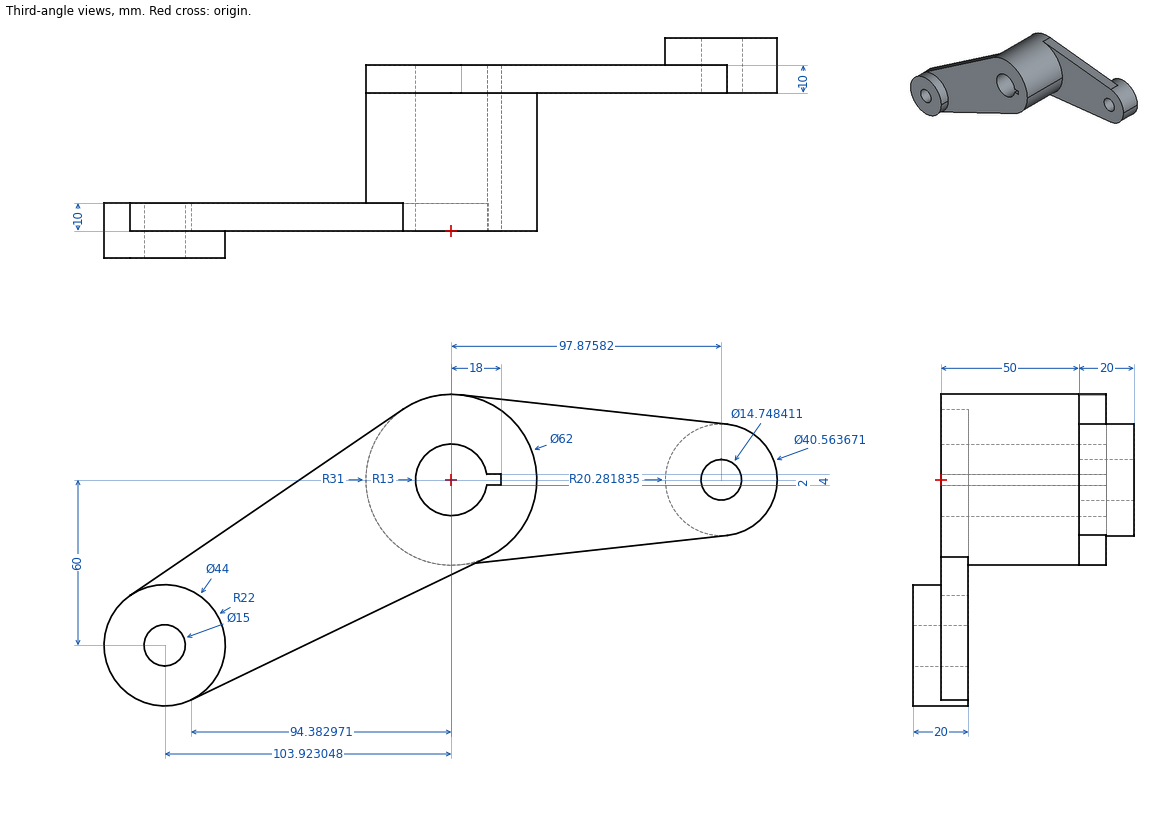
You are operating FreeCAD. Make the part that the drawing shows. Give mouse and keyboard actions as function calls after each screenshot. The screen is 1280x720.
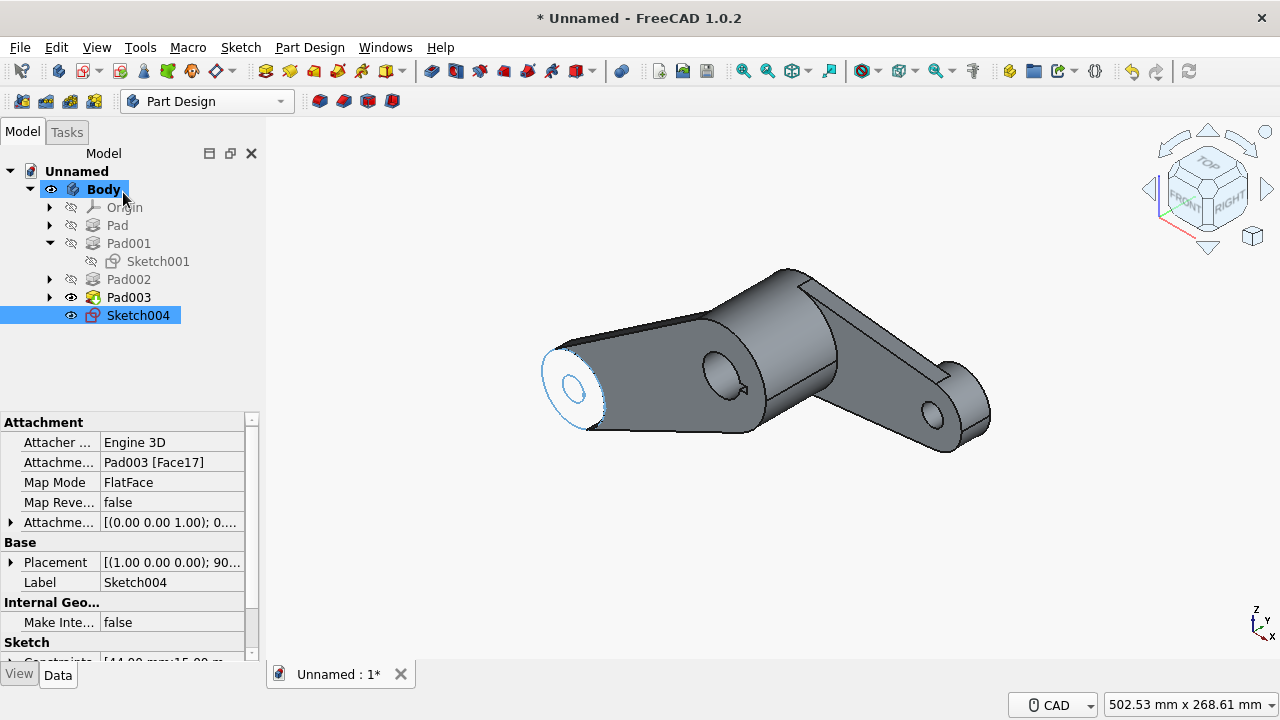
click(266, 72)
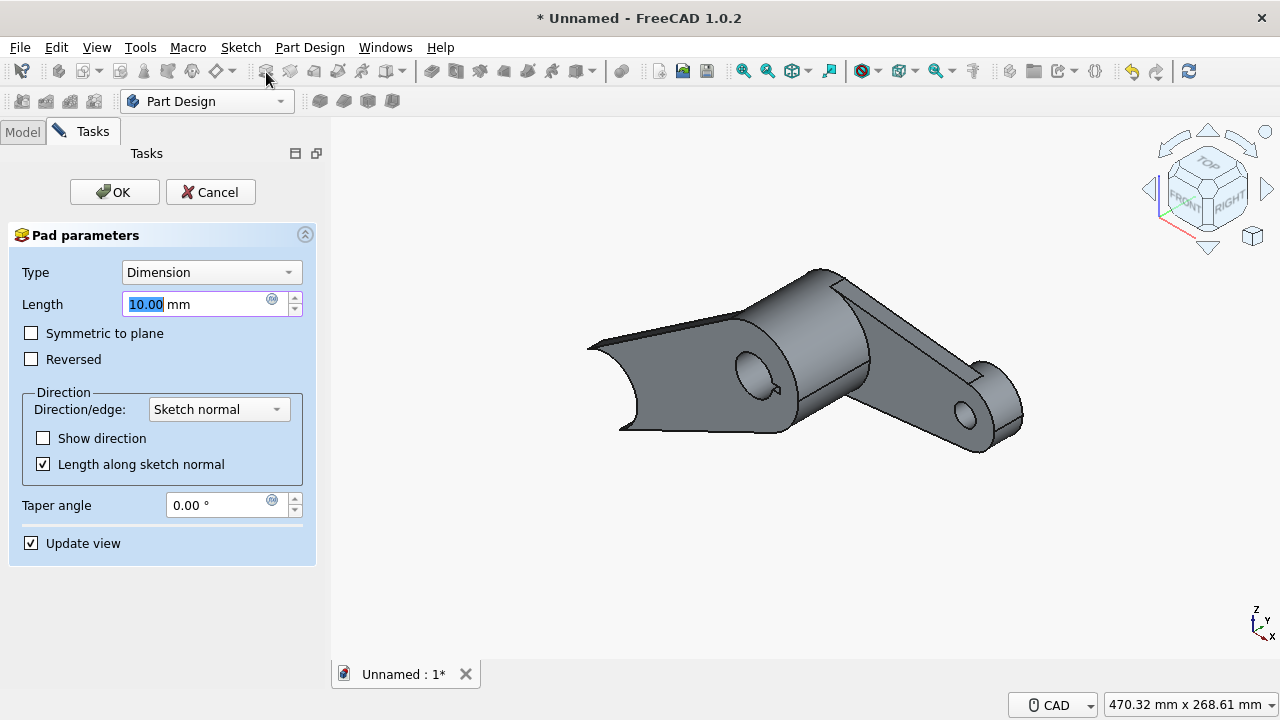
text(20)
key(Tab)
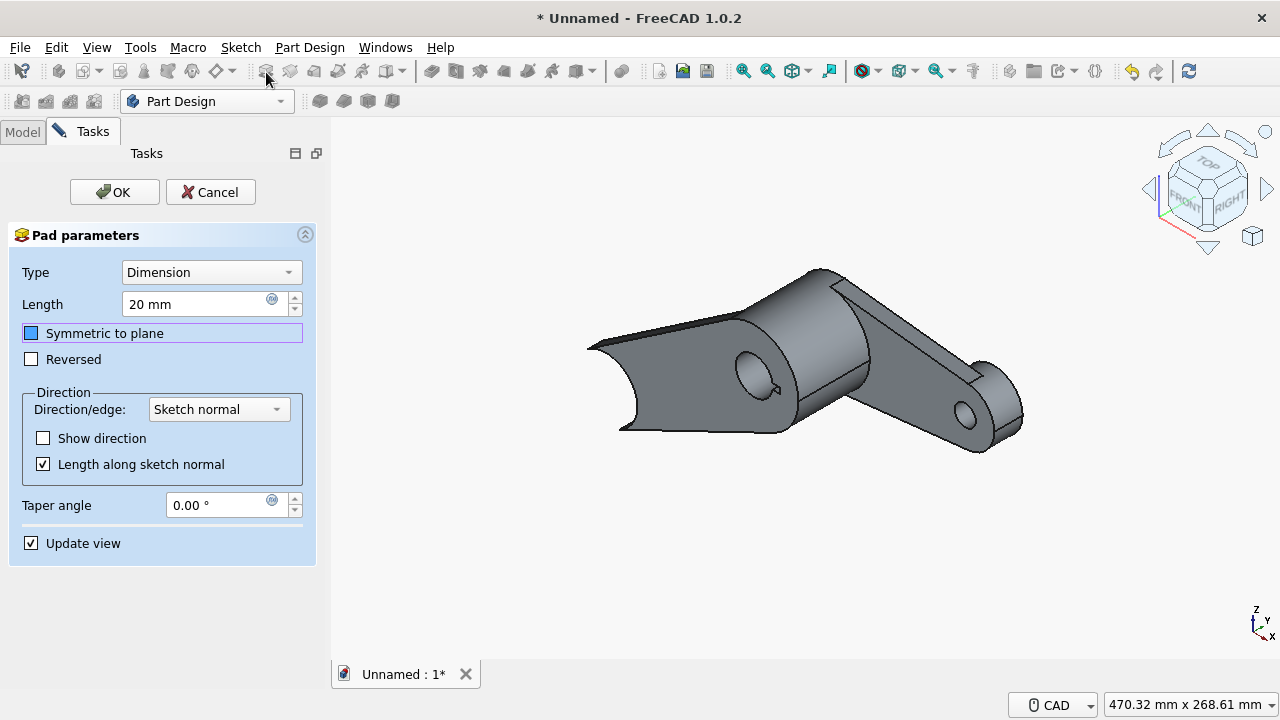
click(30, 333)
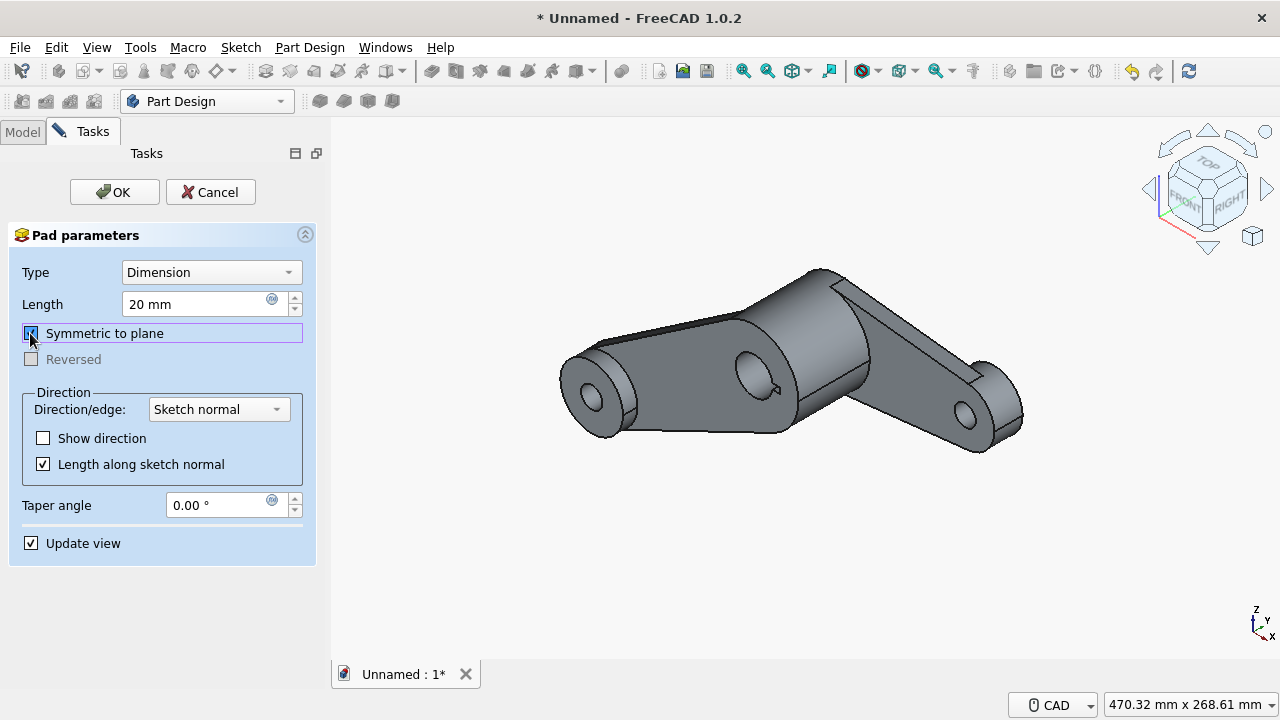
click(115, 192)